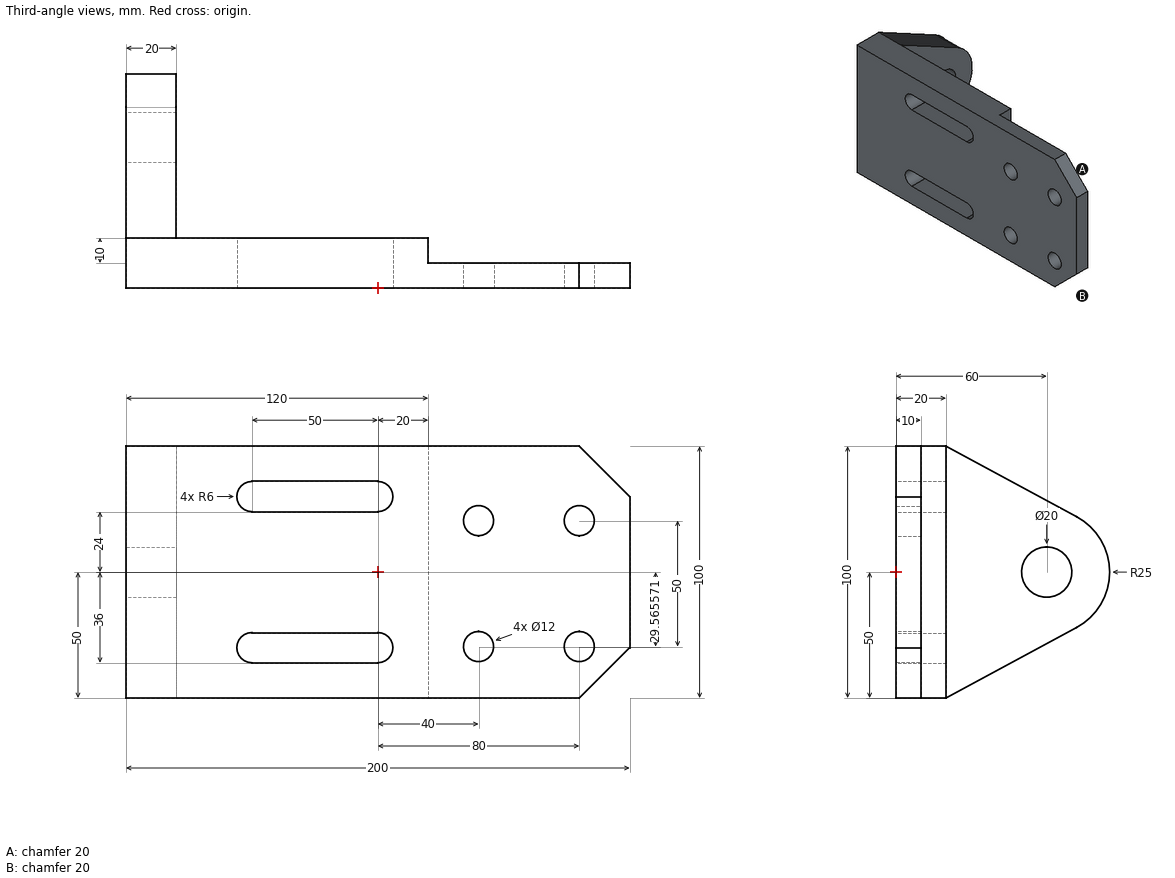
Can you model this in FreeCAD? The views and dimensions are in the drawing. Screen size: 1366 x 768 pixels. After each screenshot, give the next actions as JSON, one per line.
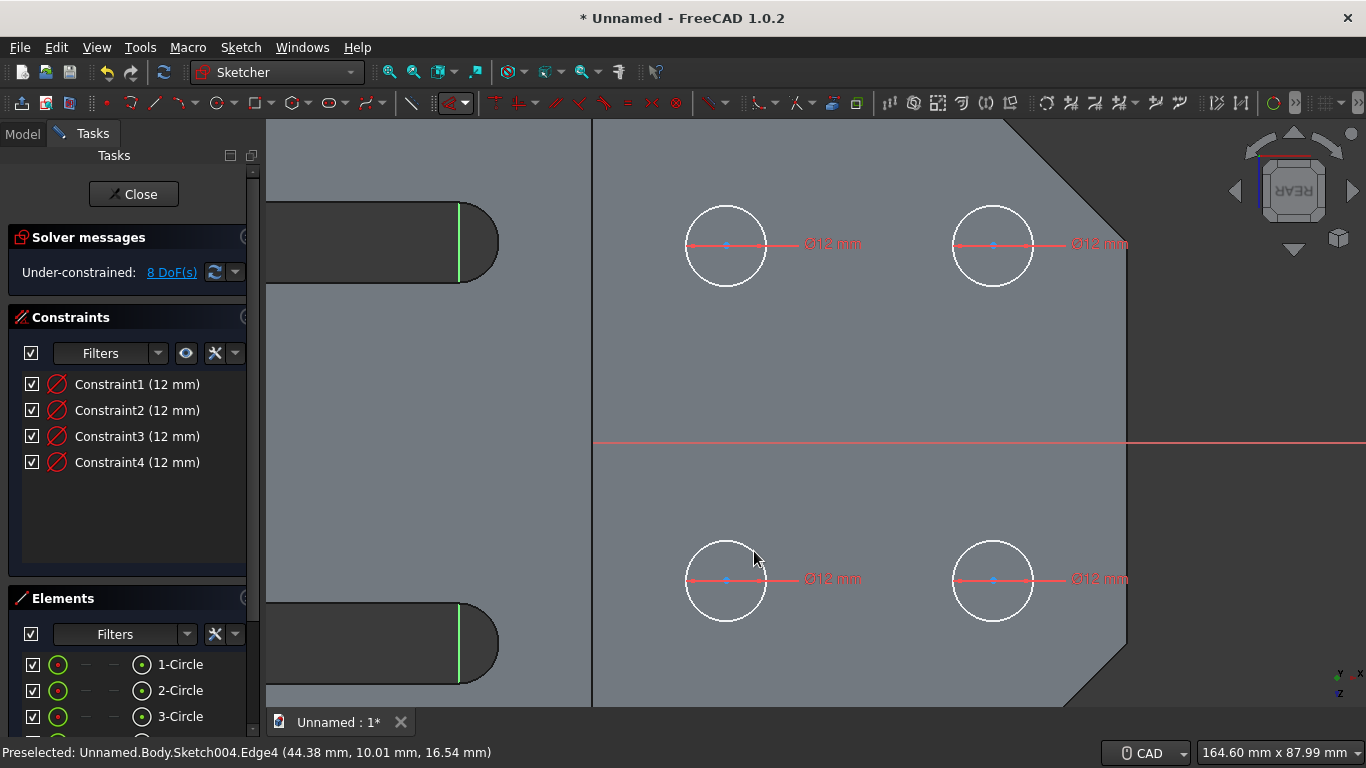
{"action": "left_click", "coordinate": [726, 246]}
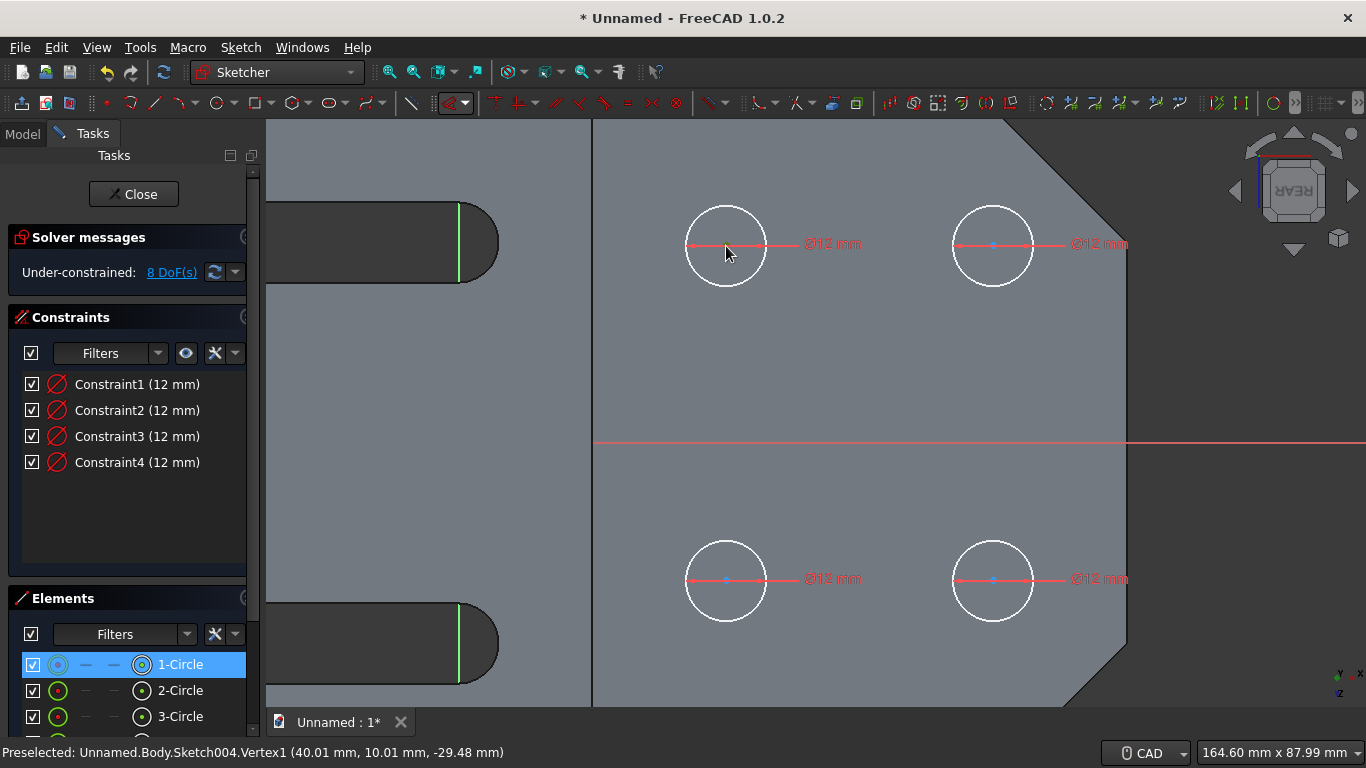
{"action": "left_click", "coordinate": [993, 246]}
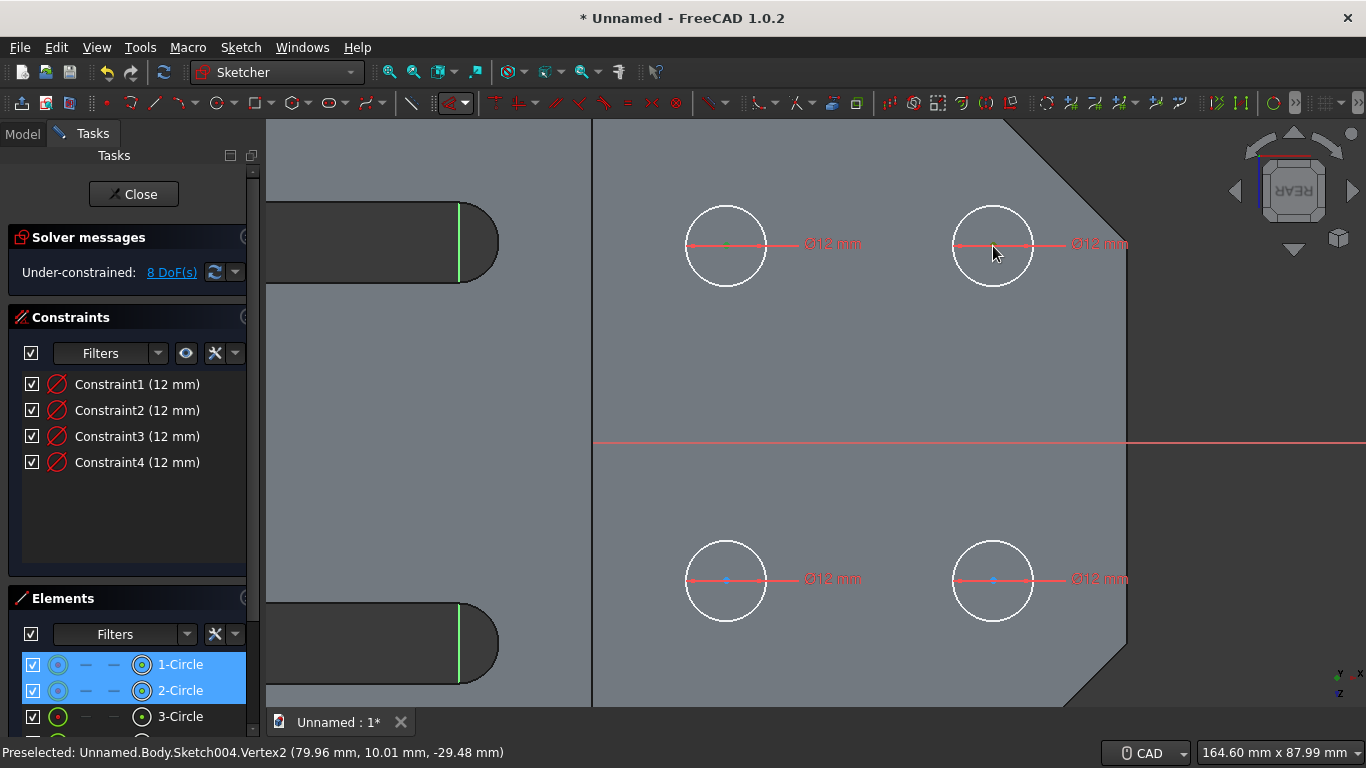
{"action": "key", "text": "h"}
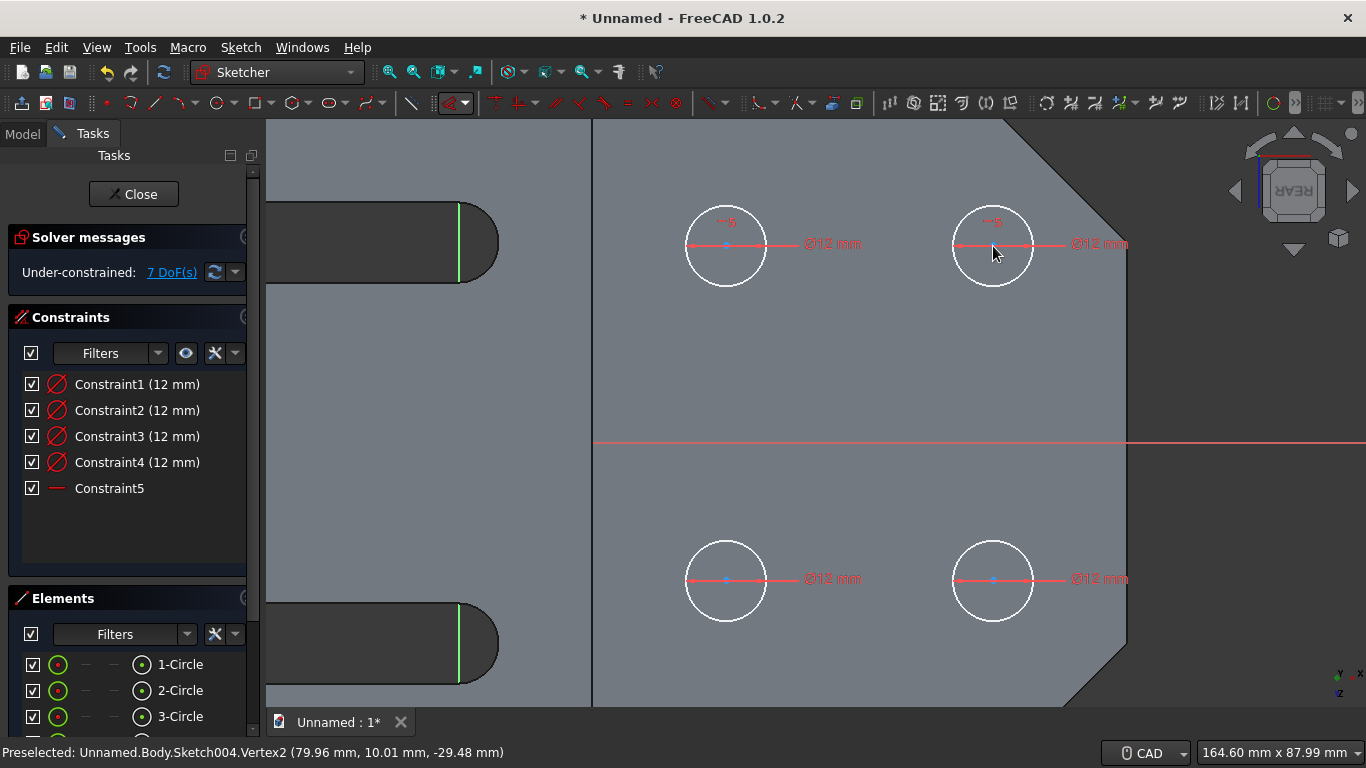
{"action": "left_click", "coordinate": [993, 246]}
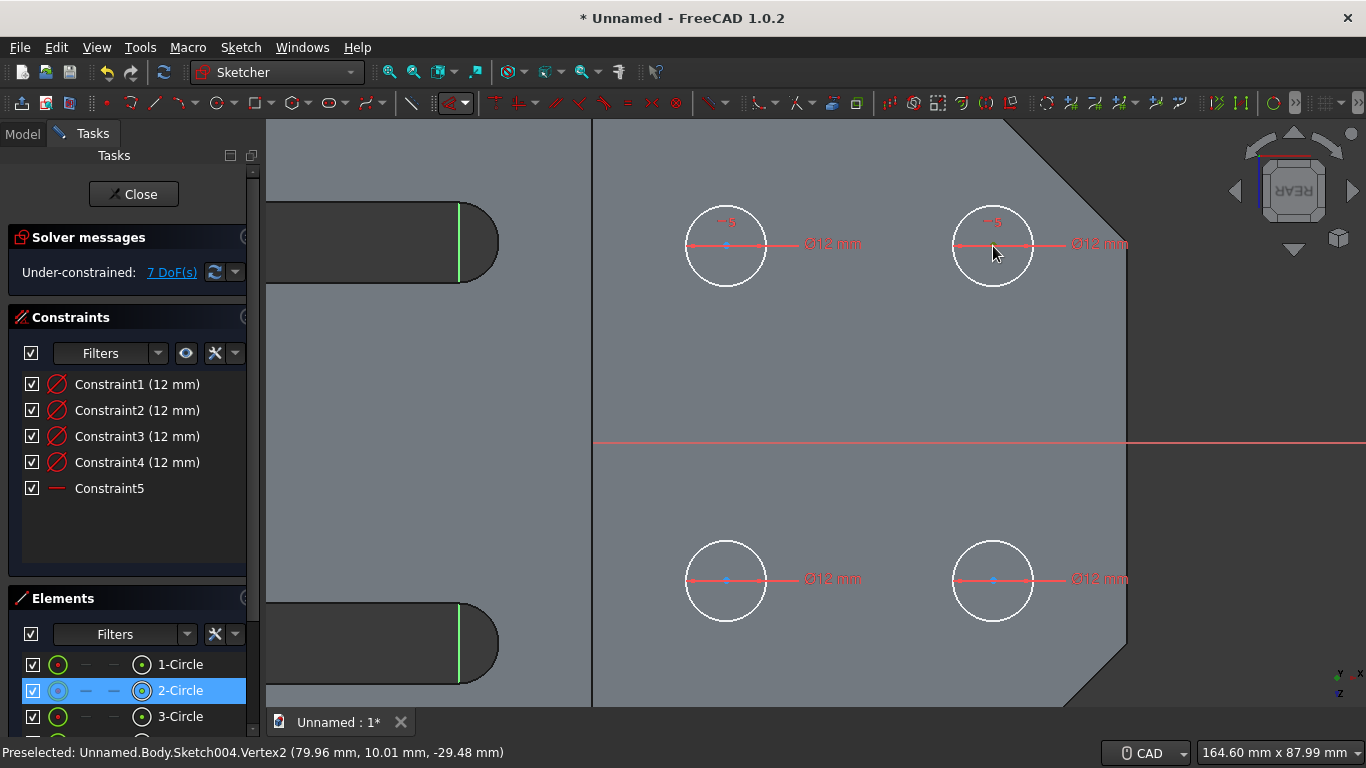
{"action": "left_click", "coordinate": [993, 581]}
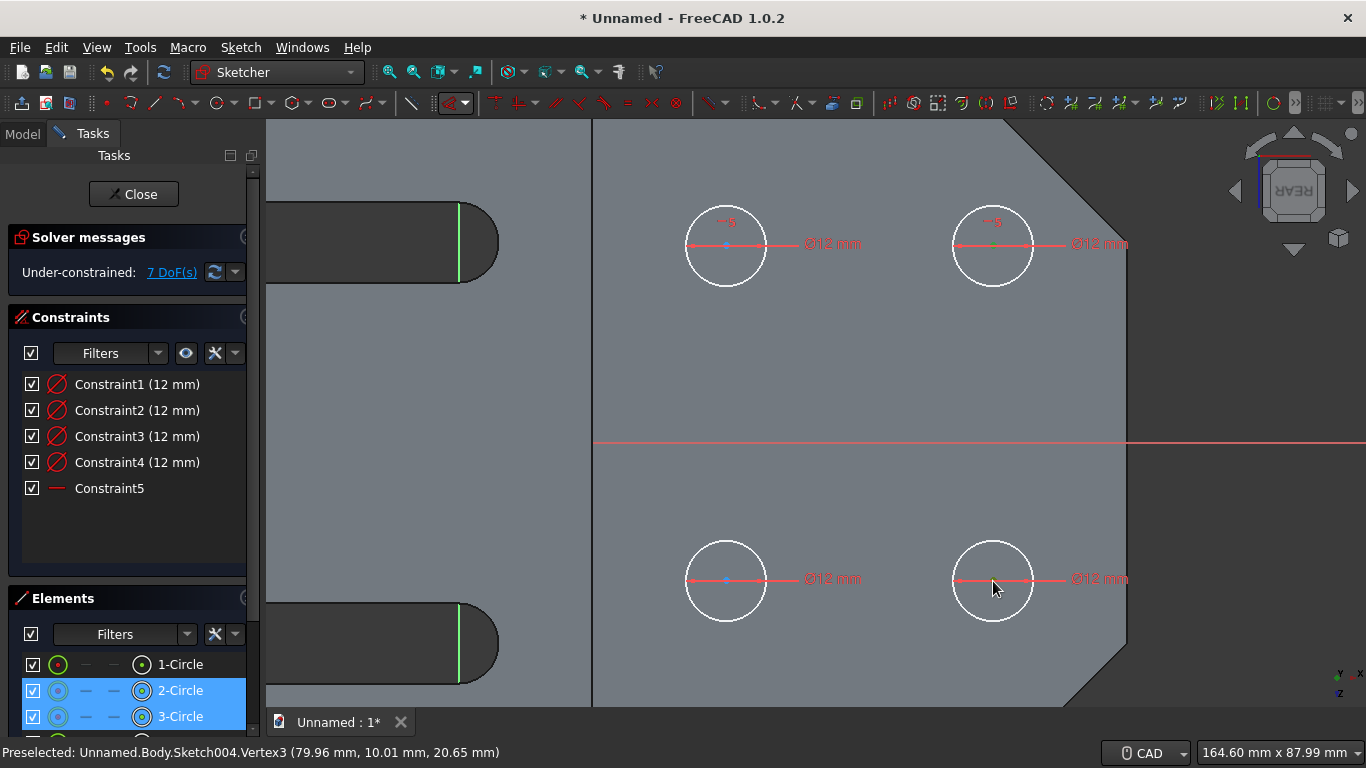
{"action": "key", "text": "v"}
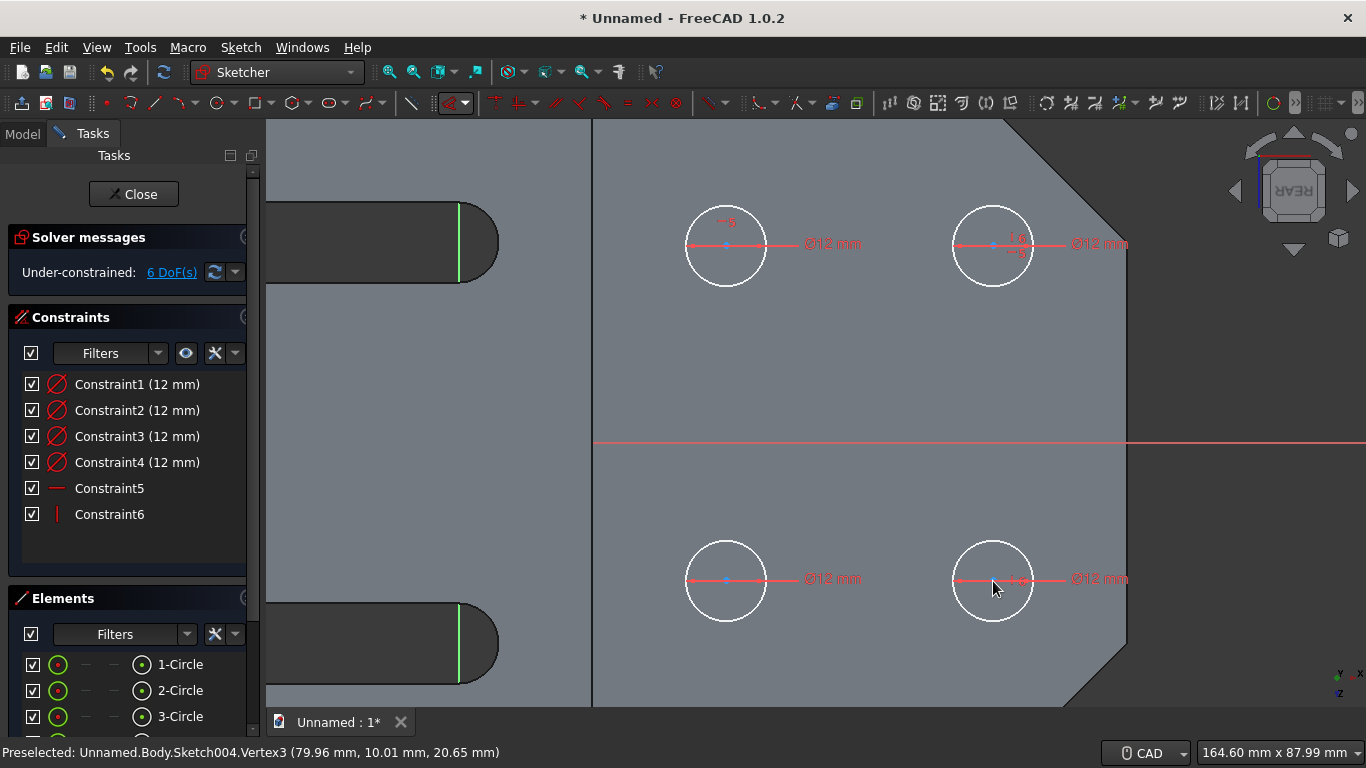
{"action": "left_click", "coordinate": [726, 246]}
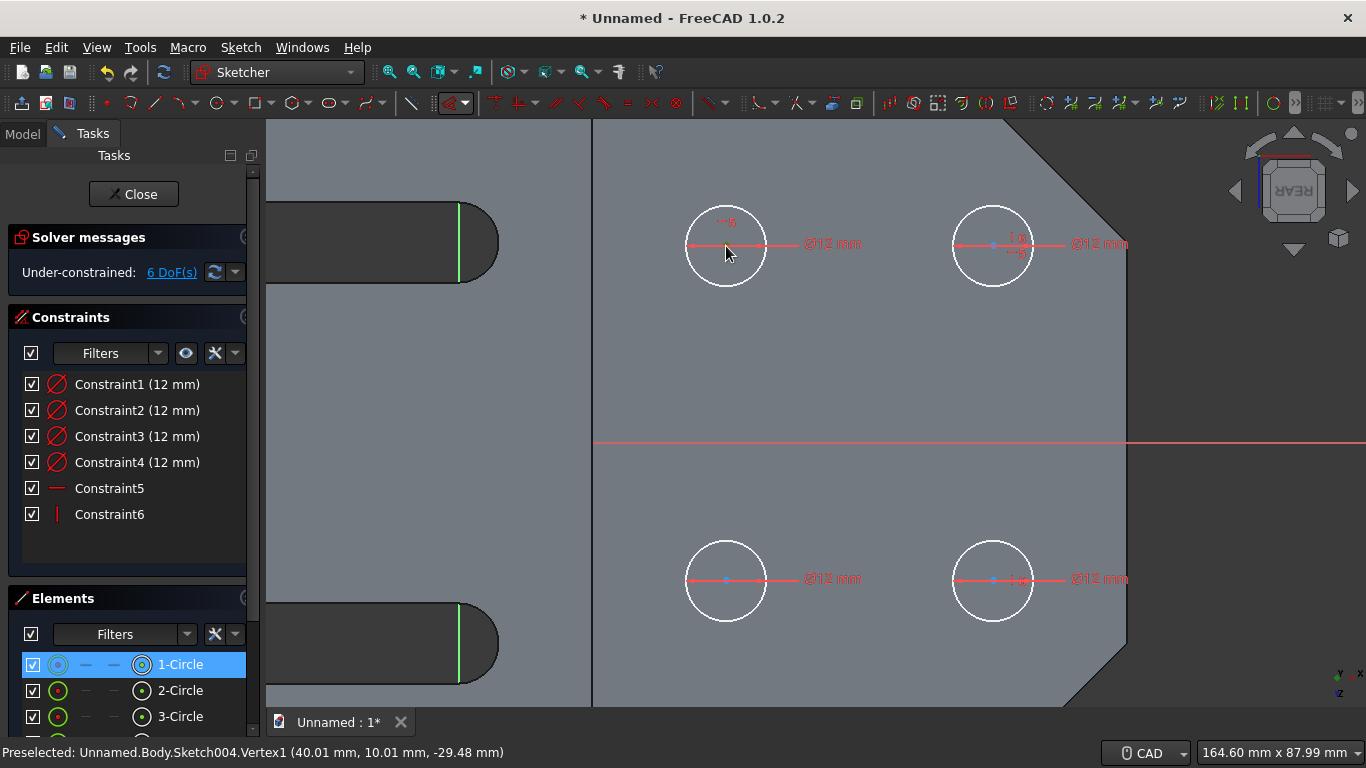
{"action": "left_click", "coordinate": [726, 581]}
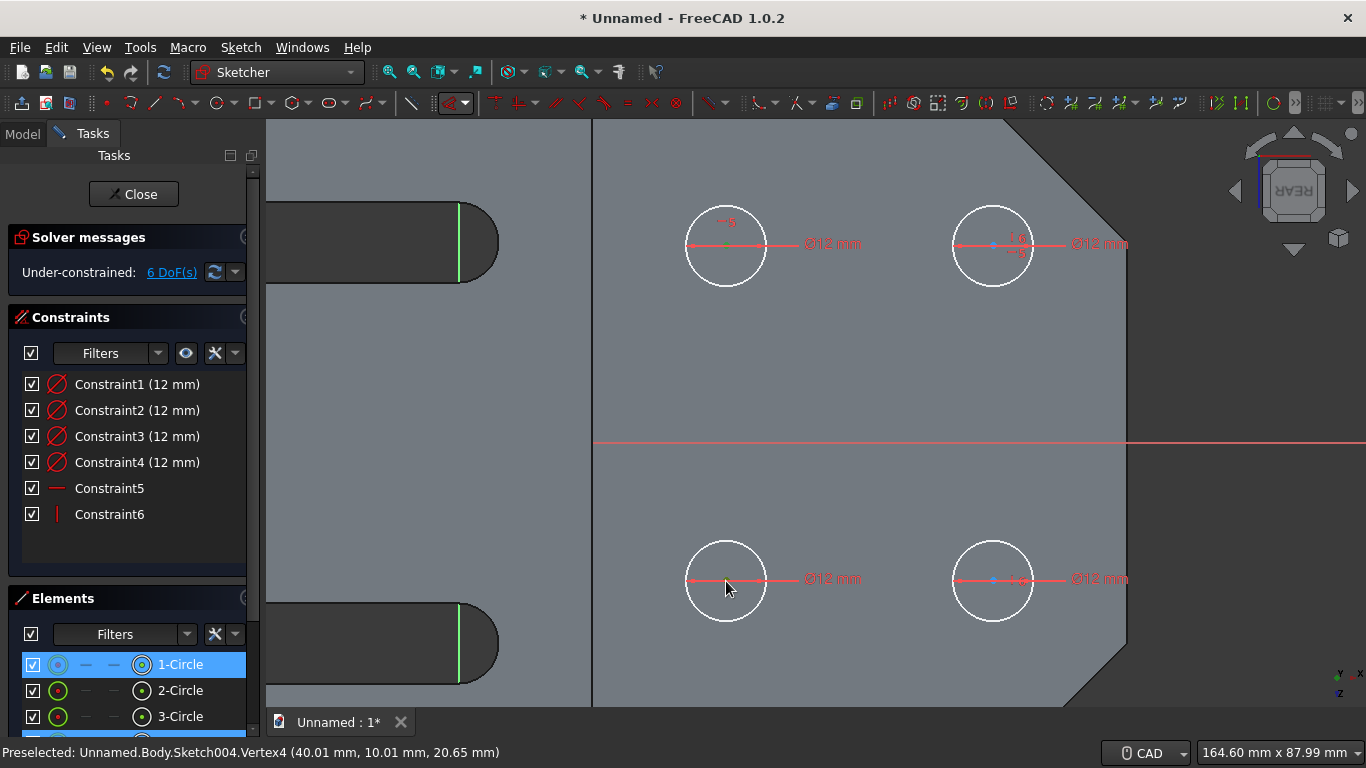
{"action": "key", "text": "v"}